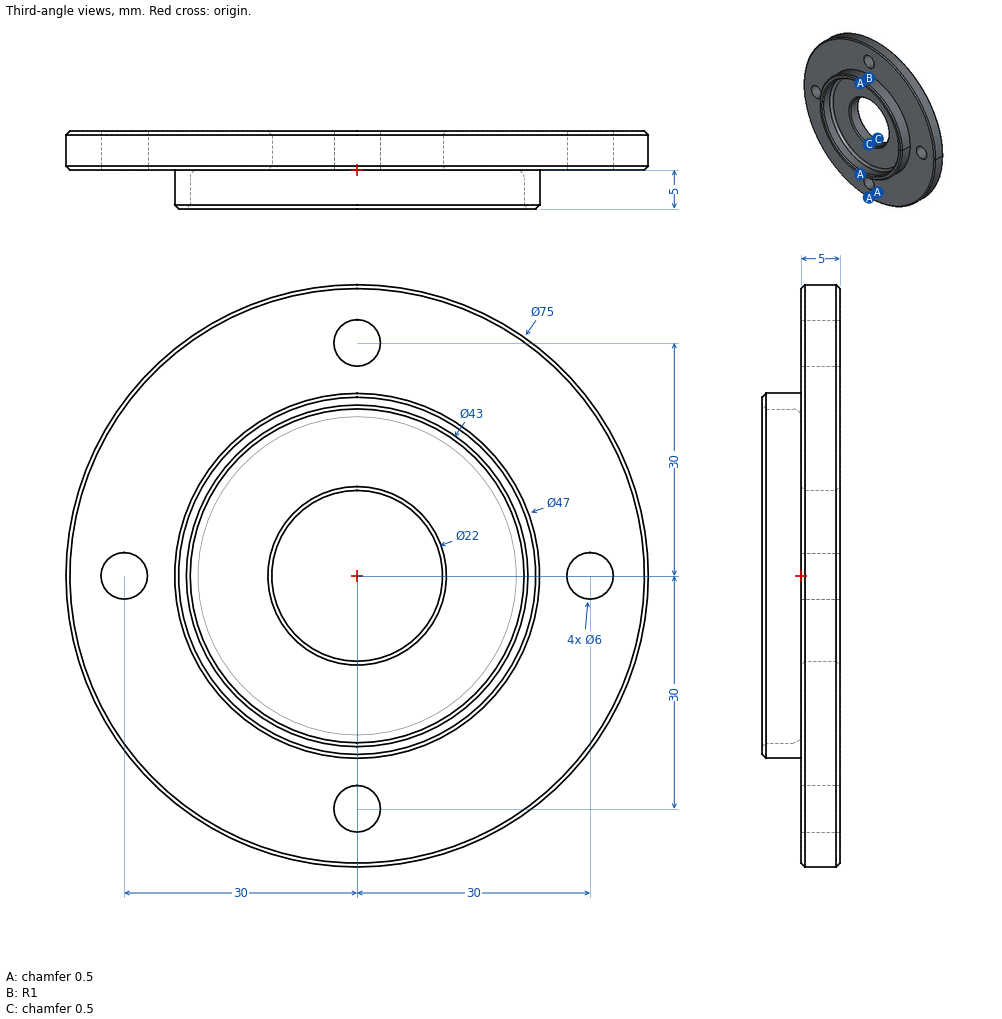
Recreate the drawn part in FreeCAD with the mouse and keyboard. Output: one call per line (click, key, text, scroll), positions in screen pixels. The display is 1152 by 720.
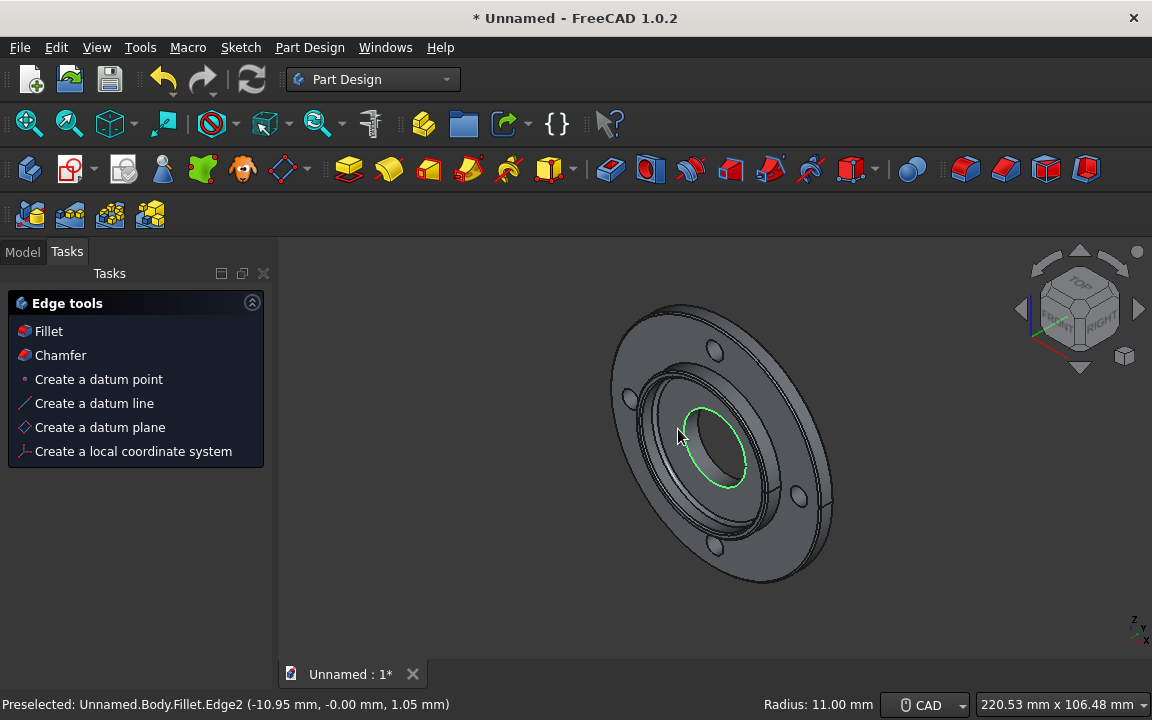
key(2)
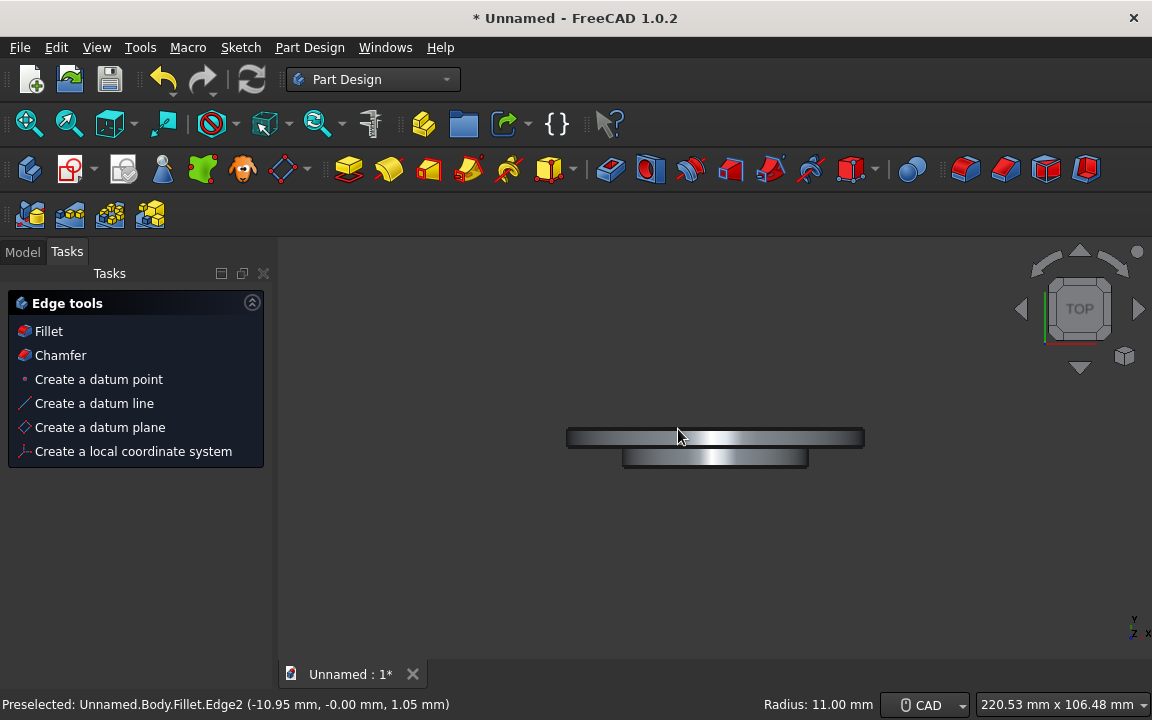
key(v)
key(f)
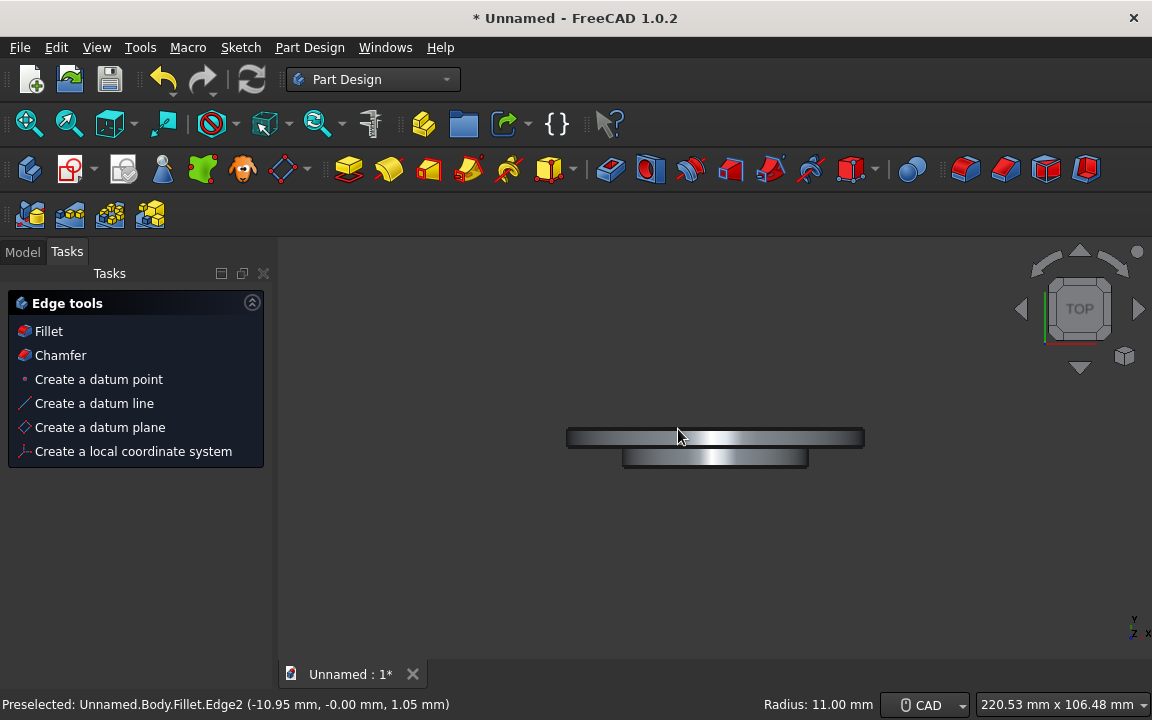
key(0)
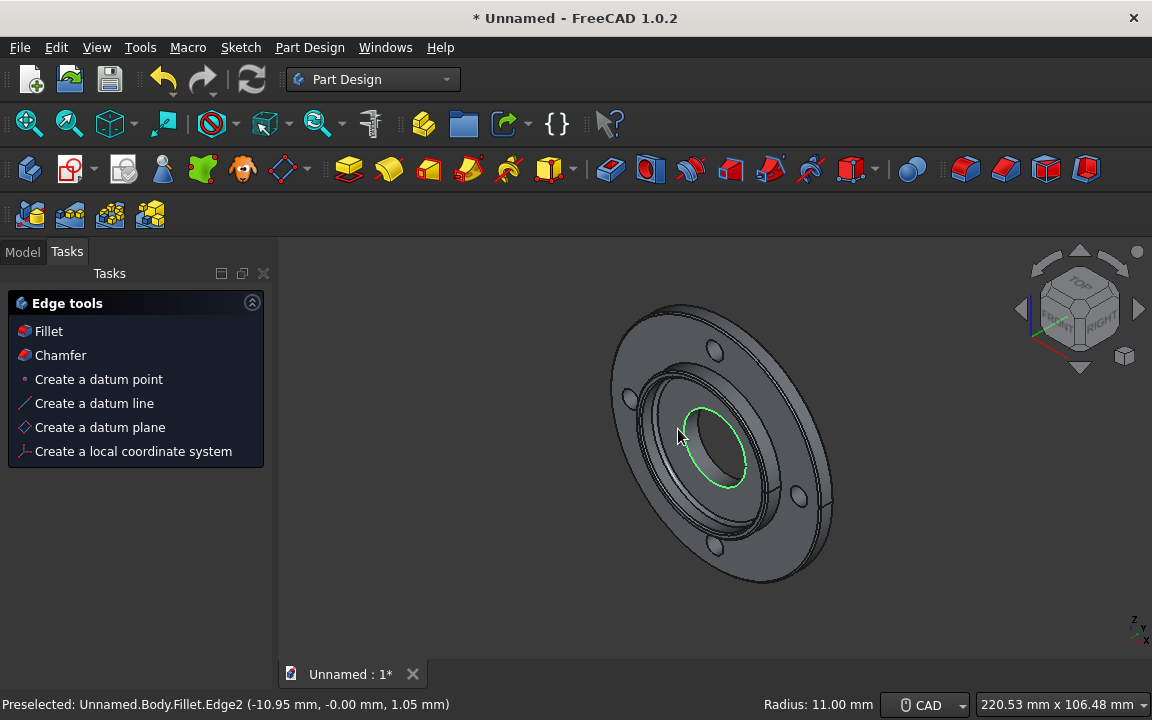
key(1)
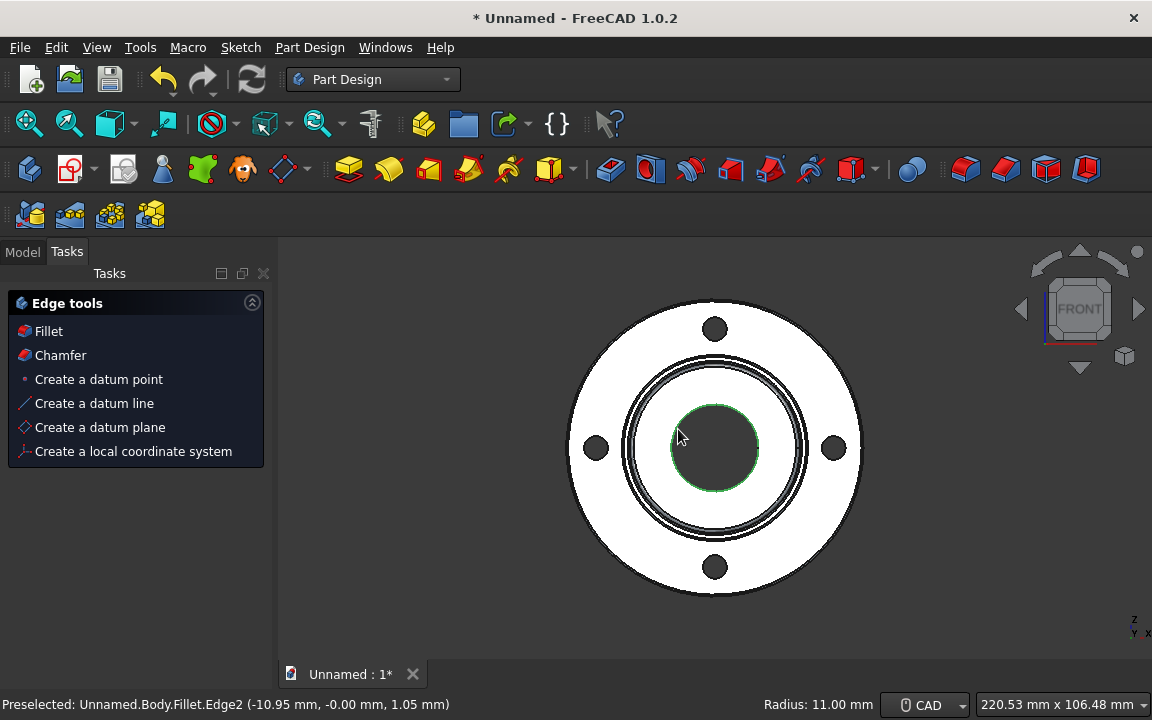
key(3)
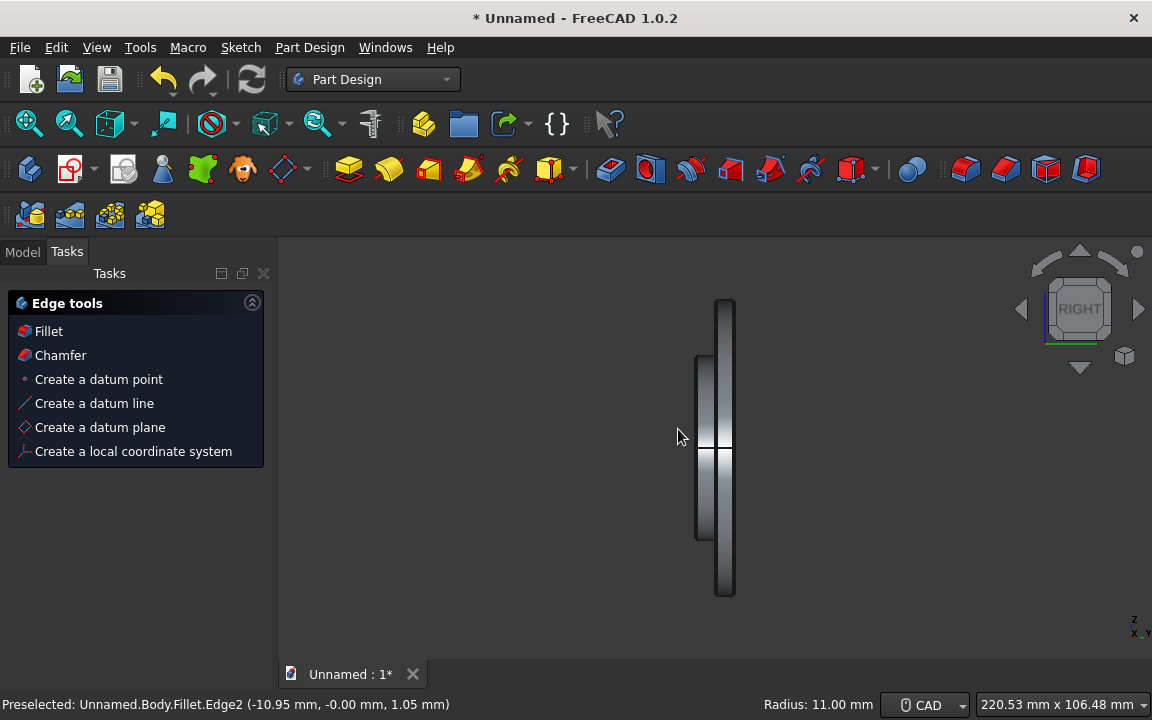
key(5)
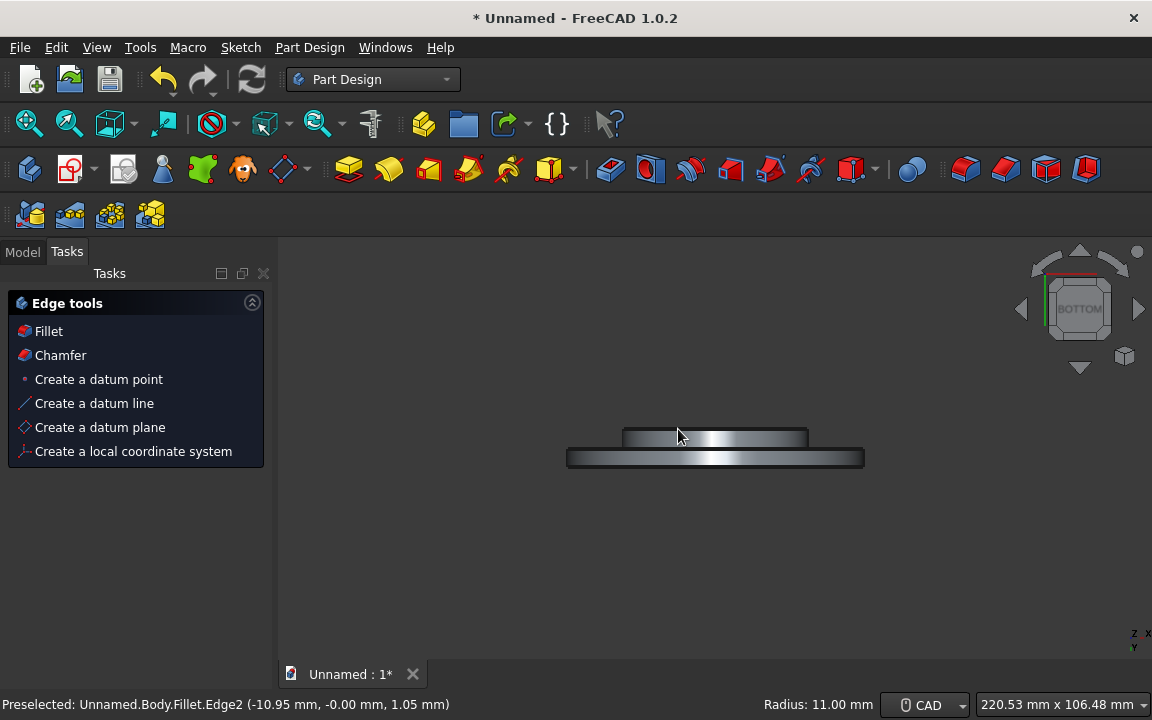
click(30, 124)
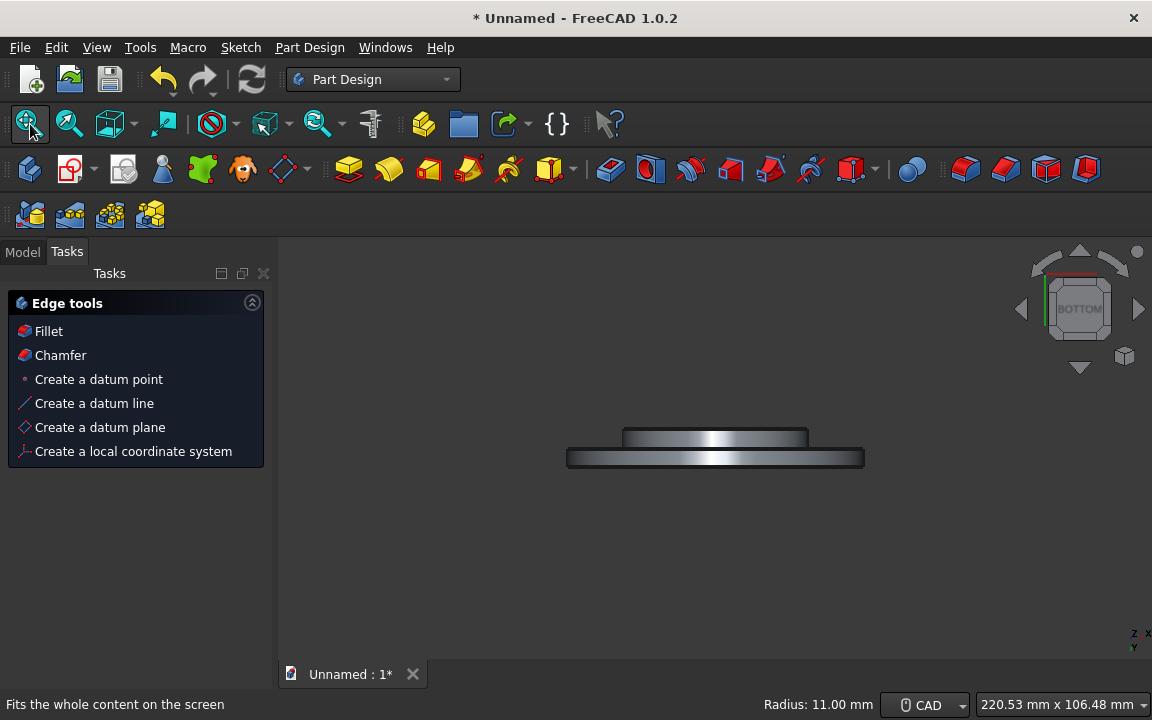
key(4)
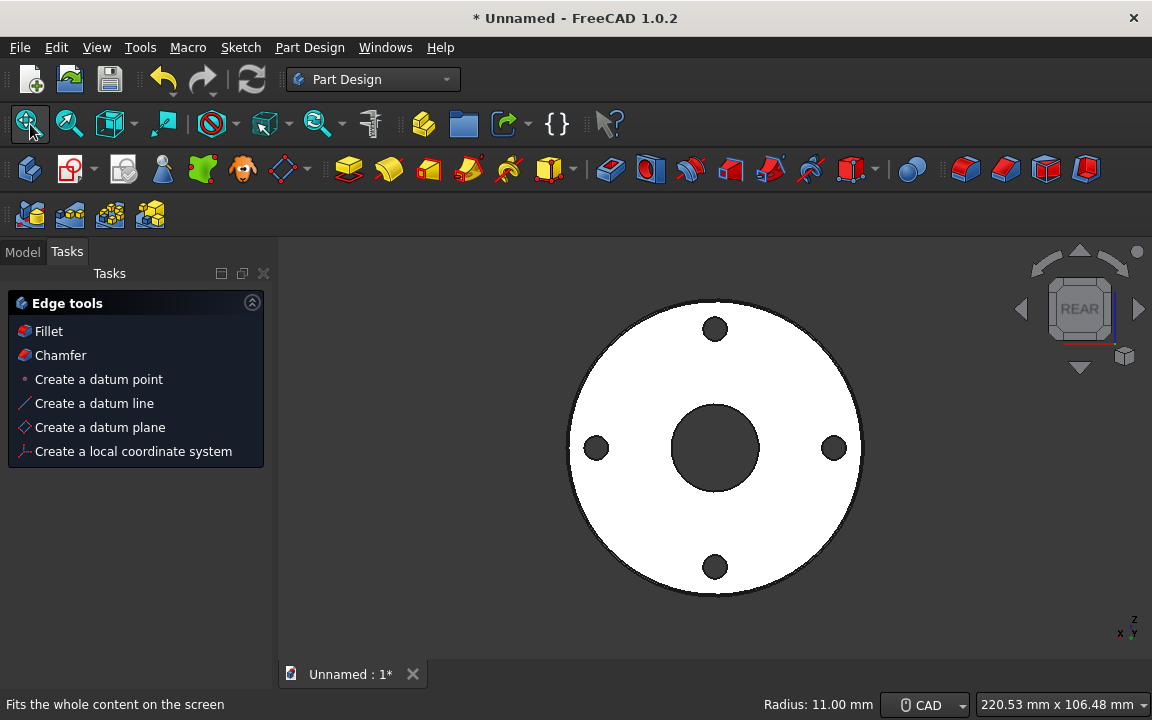
click(759, 447, ctrl)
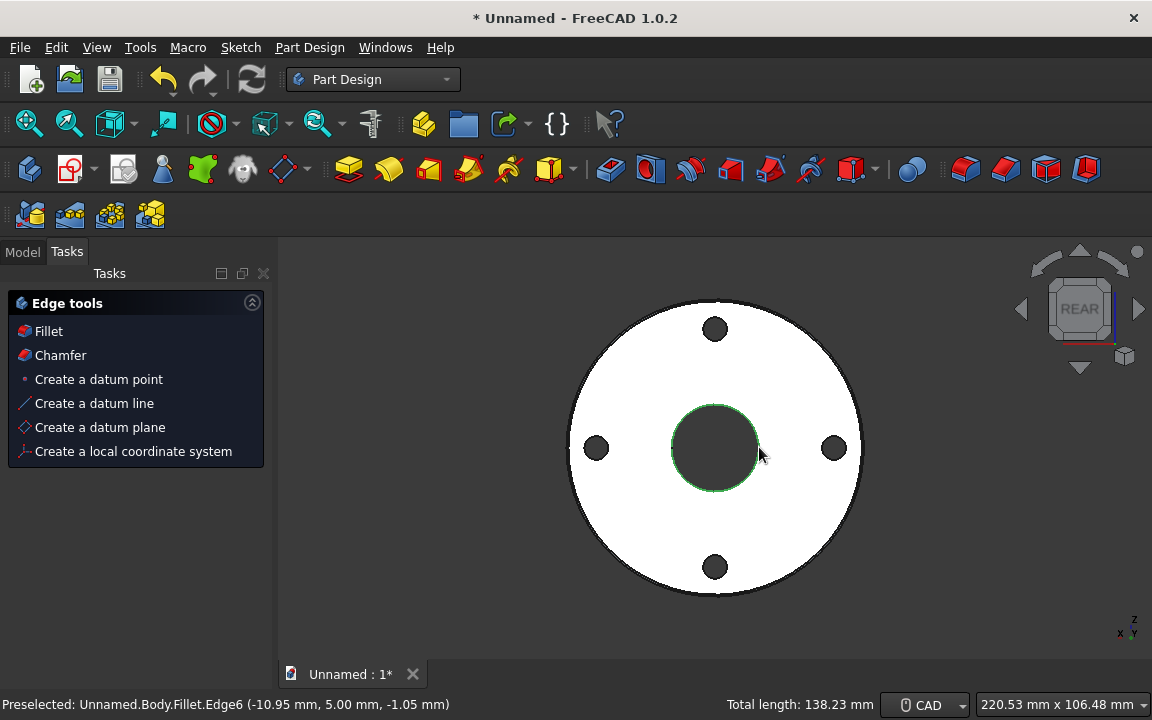
click(1006, 170)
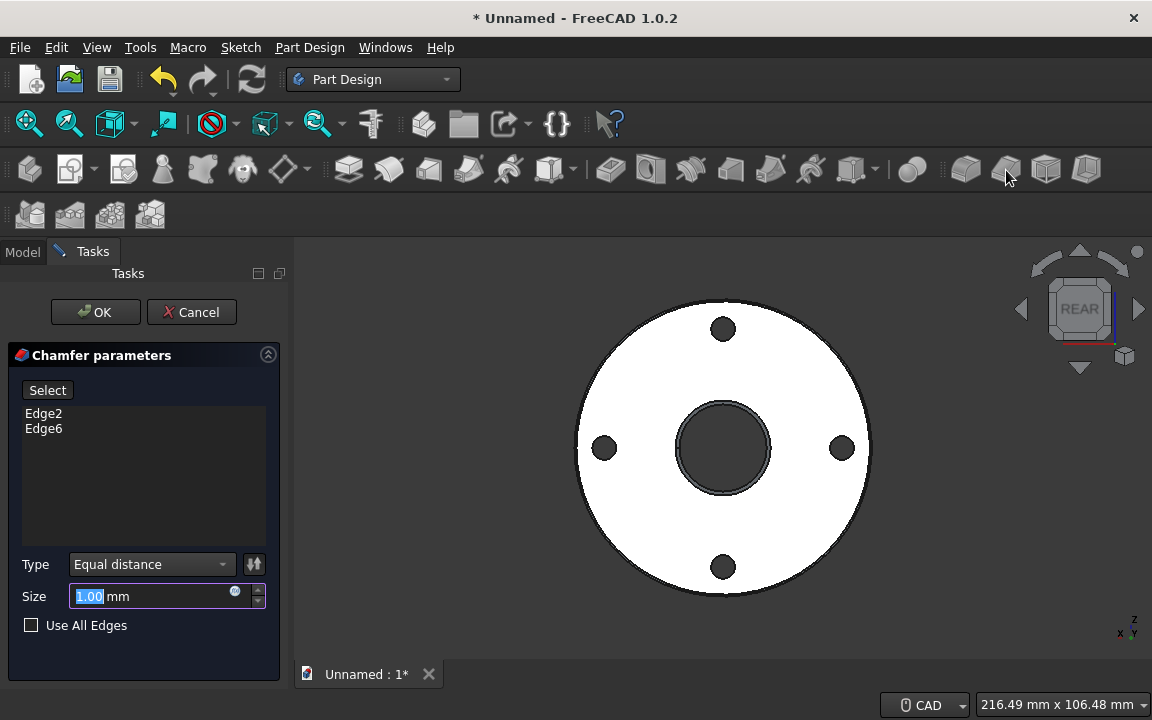
text(0.5)
key(Tab)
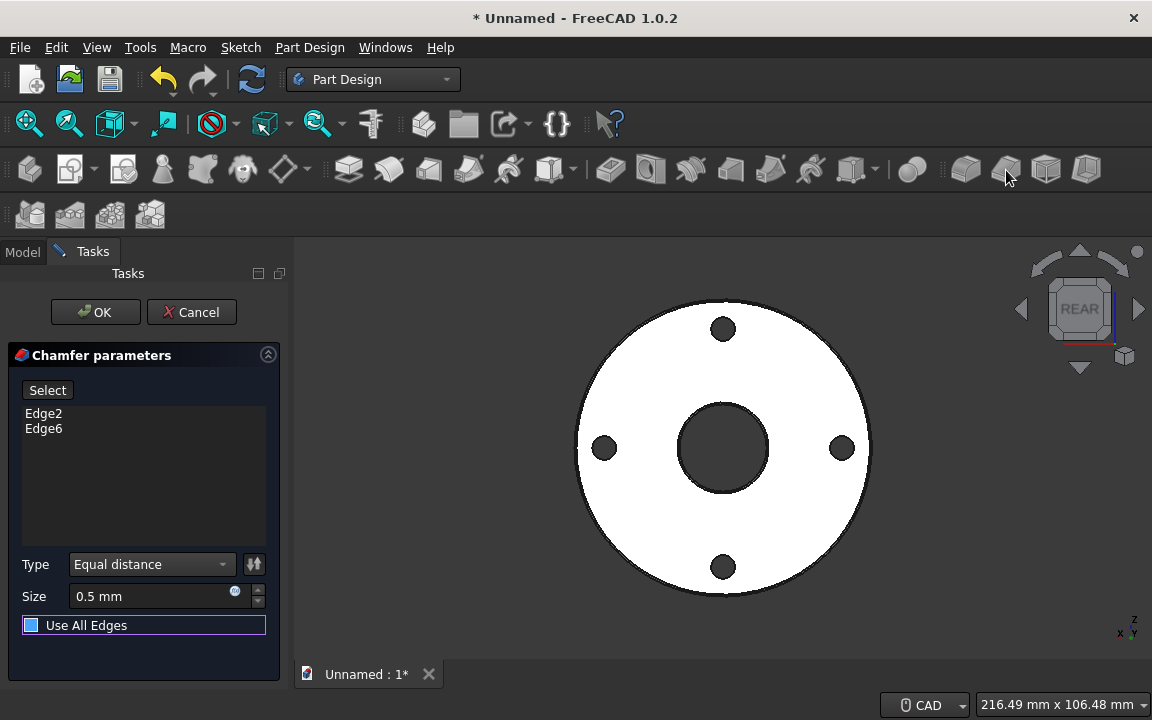
click(96, 312)